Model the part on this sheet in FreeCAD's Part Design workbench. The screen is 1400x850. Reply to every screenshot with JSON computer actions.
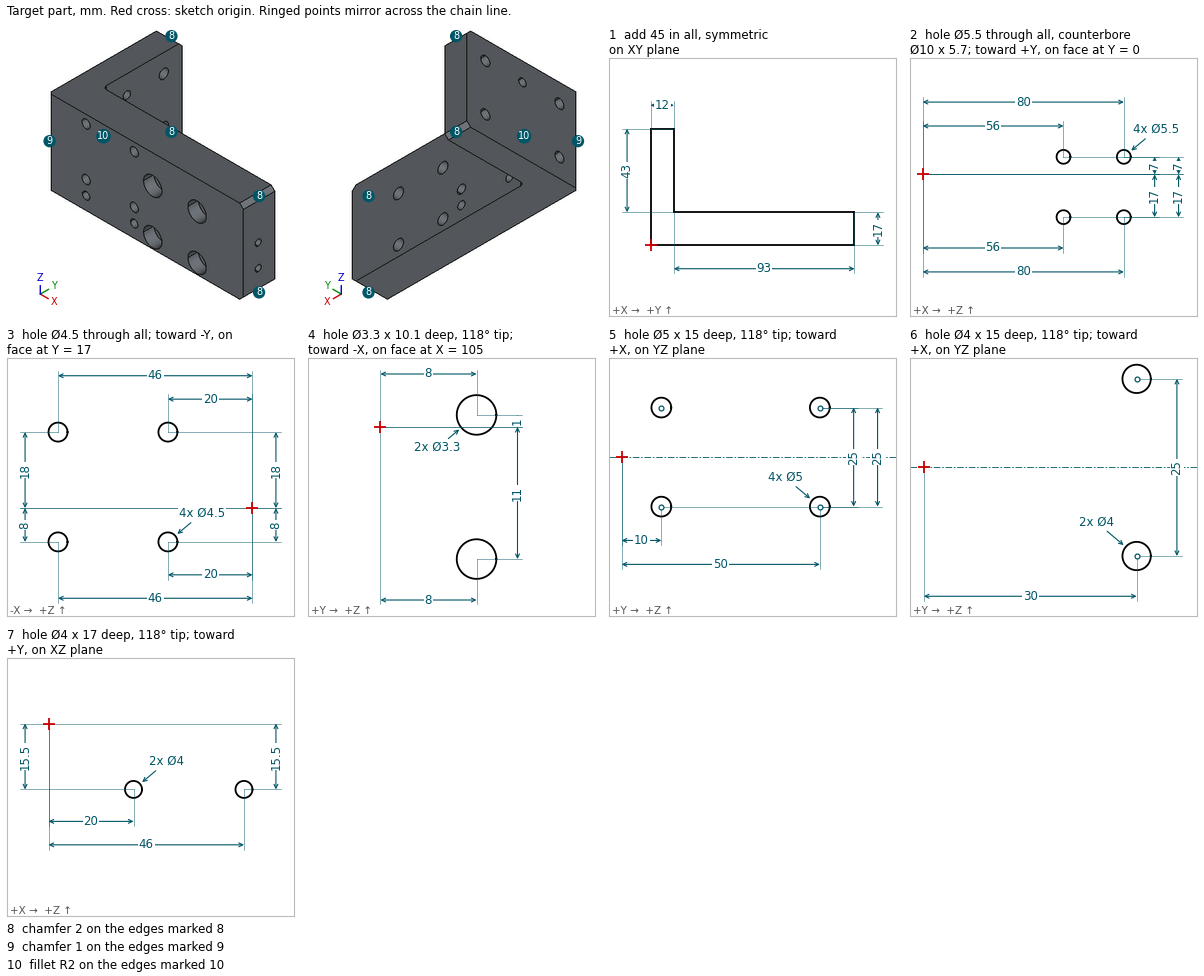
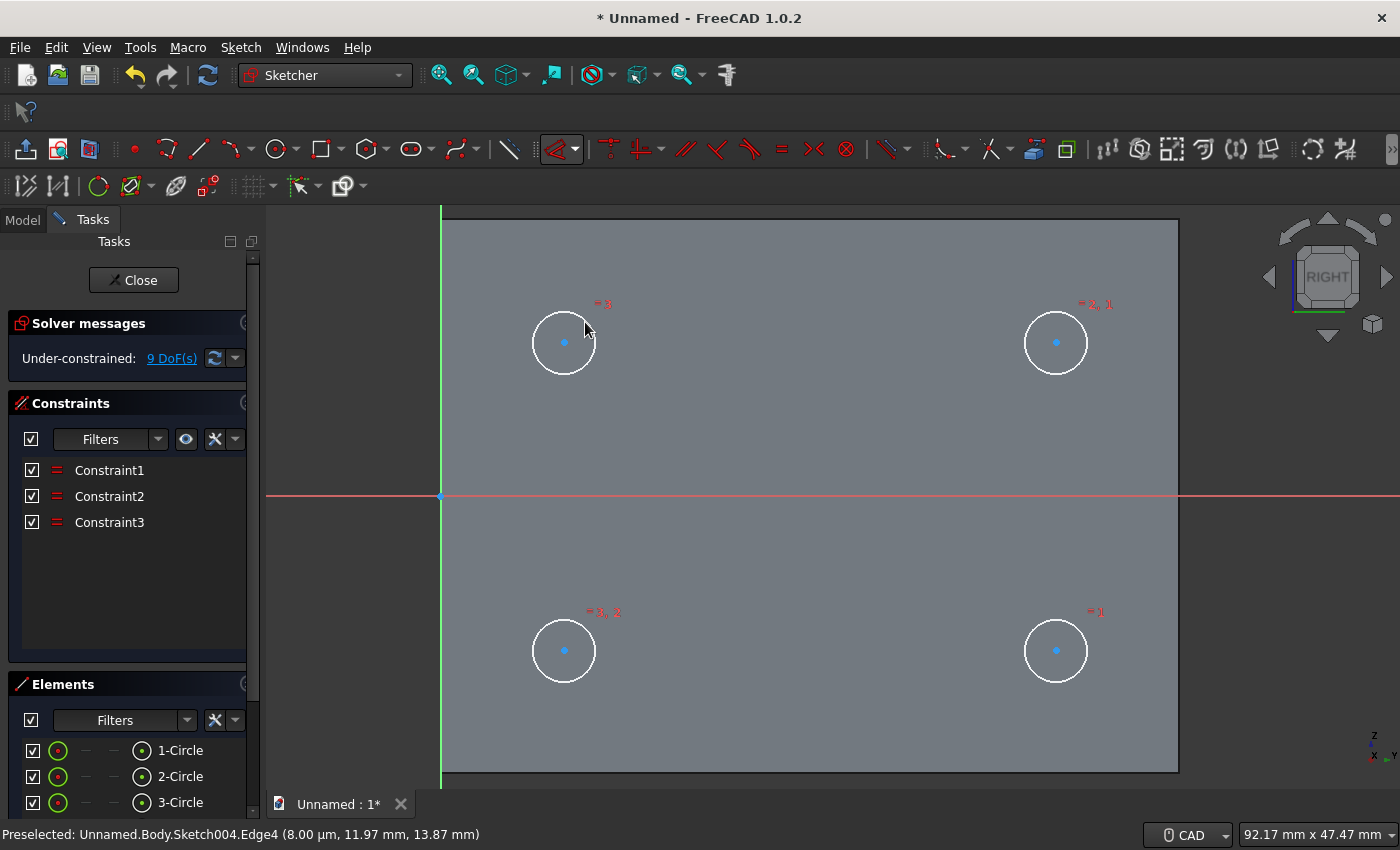
{"action": "left_click", "coordinate": [1056, 651]}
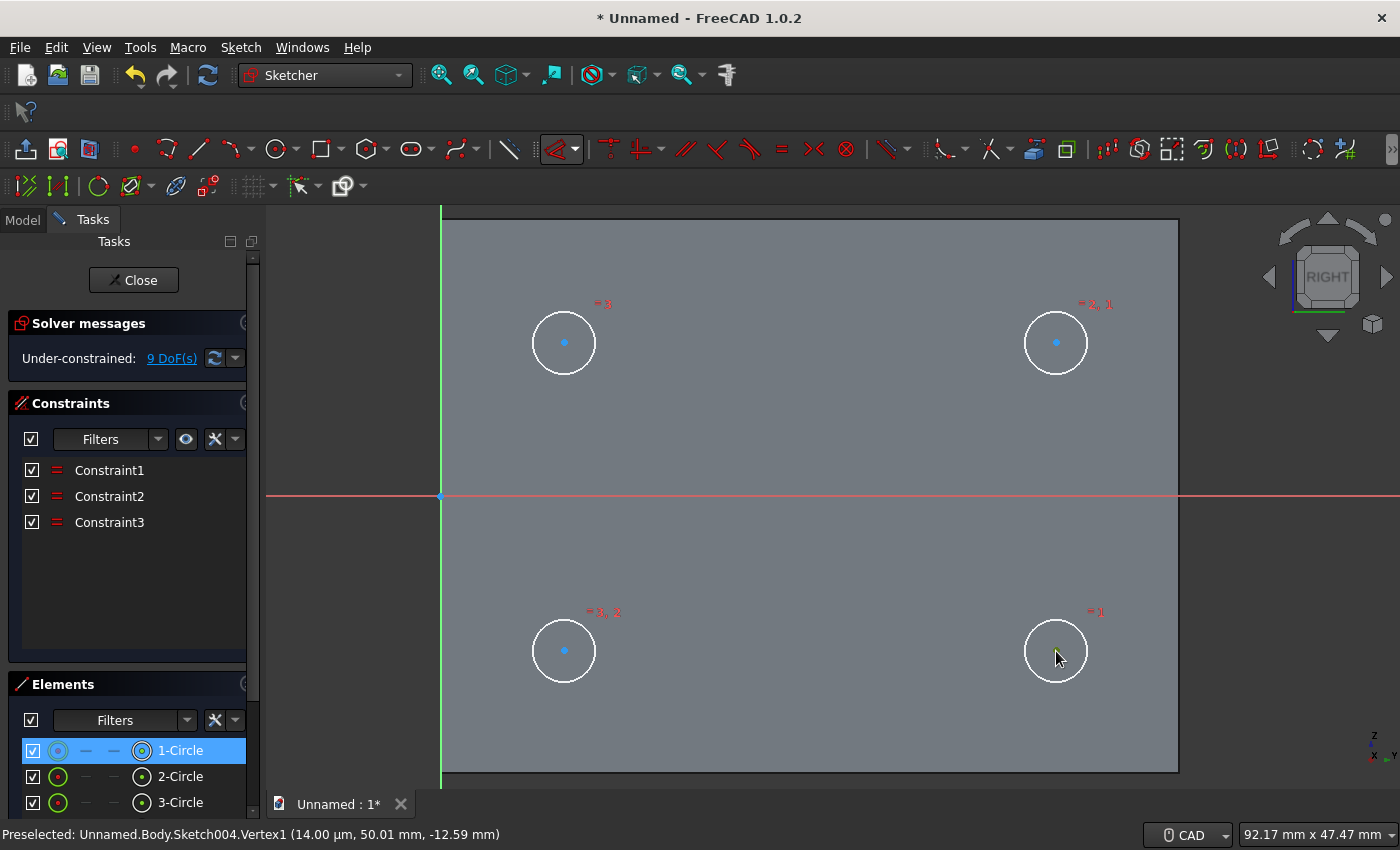
{"action": "left_click", "coordinate": [1056, 343]}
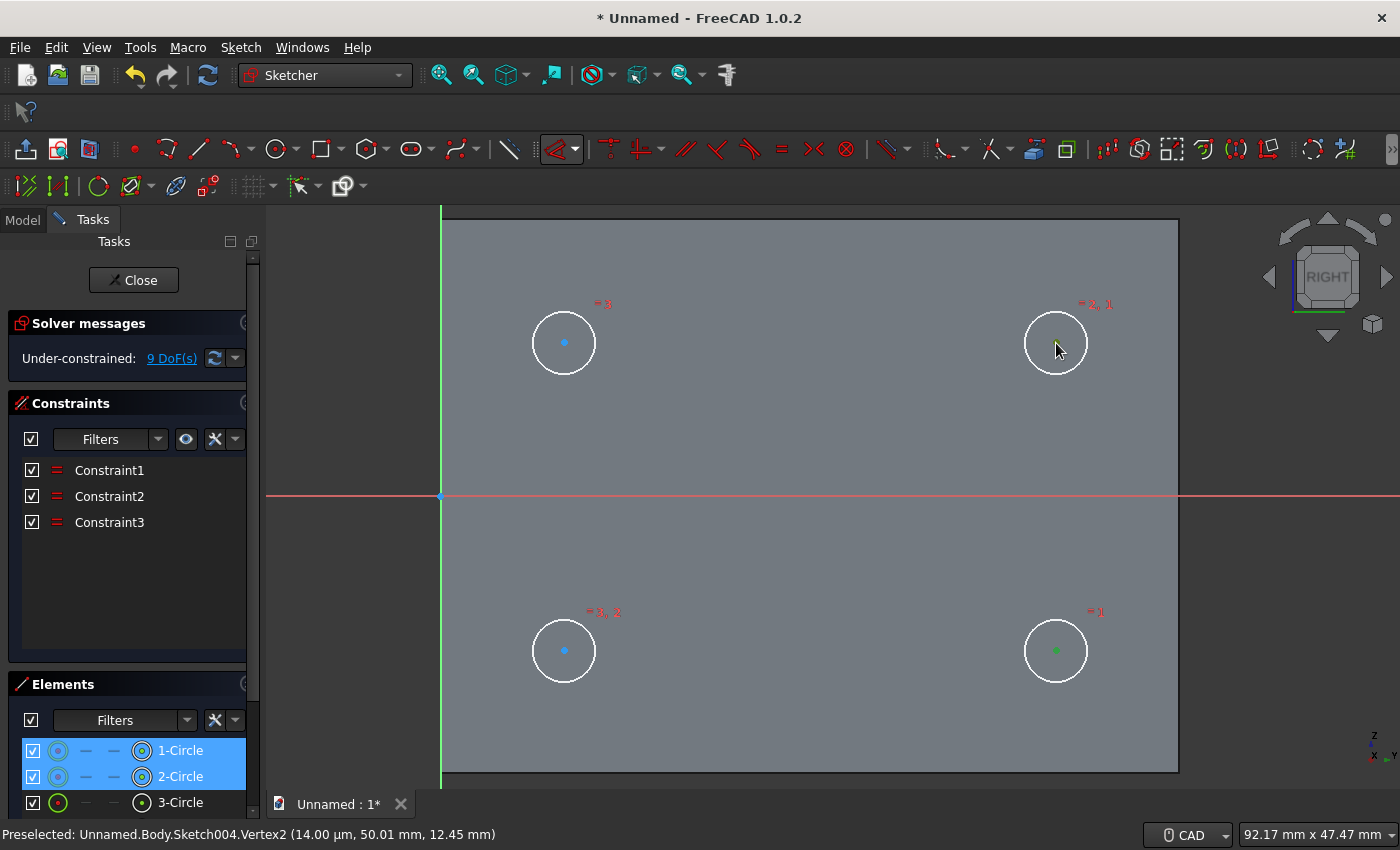
{"action": "left_click", "coordinate": [361, 496]}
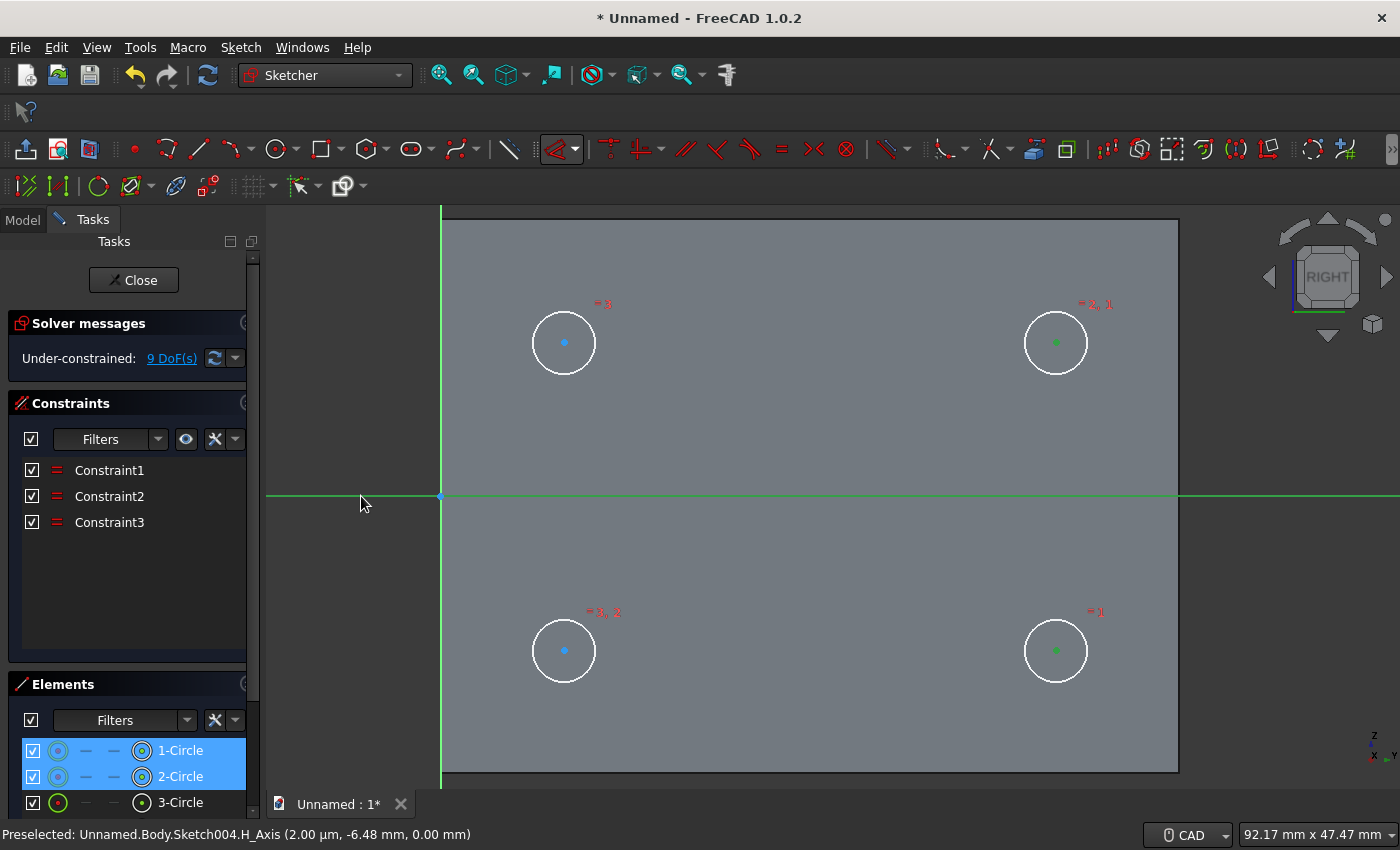
{"action": "key", "text": "s"}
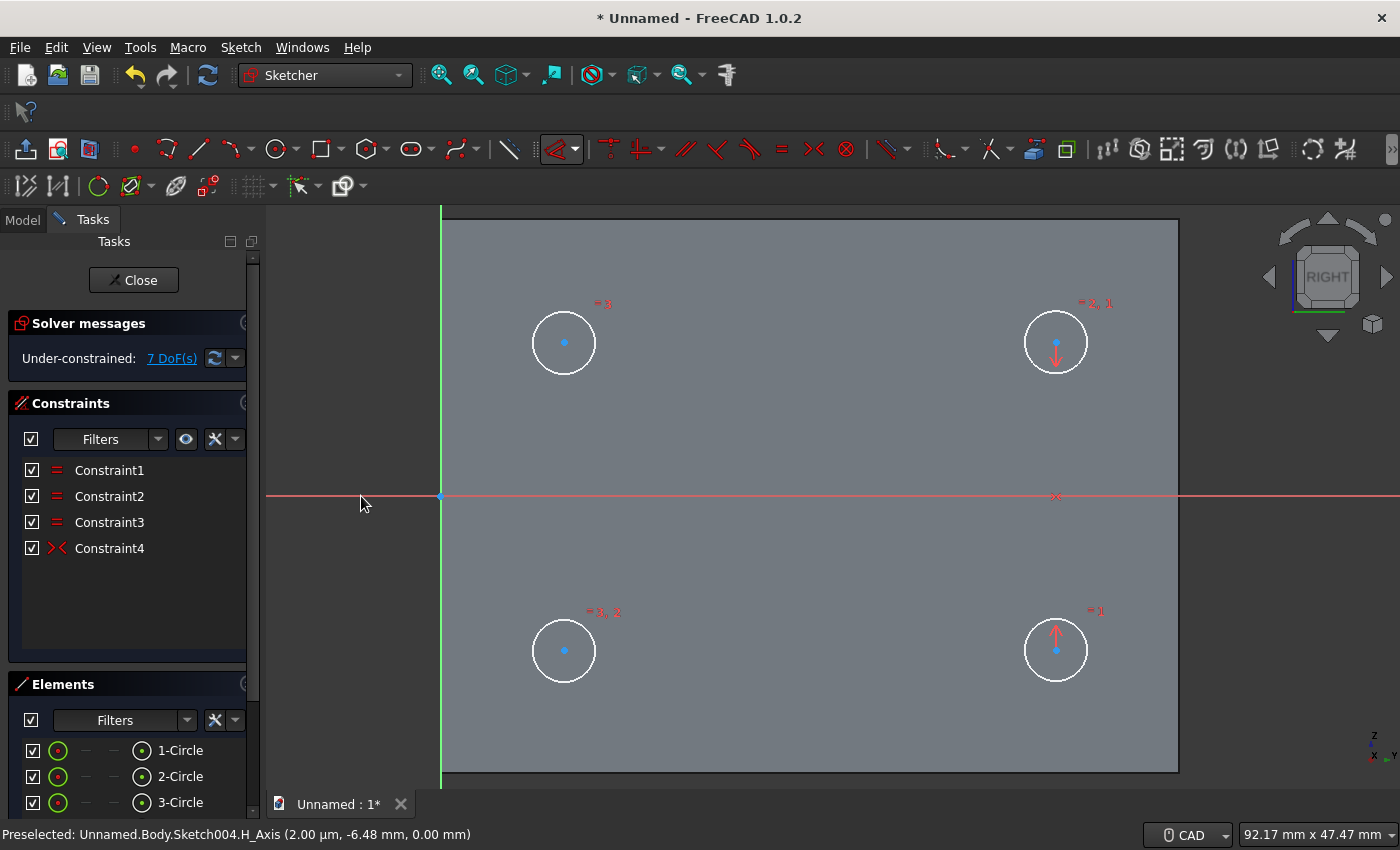
{"action": "left_click", "coordinate": [564, 651]}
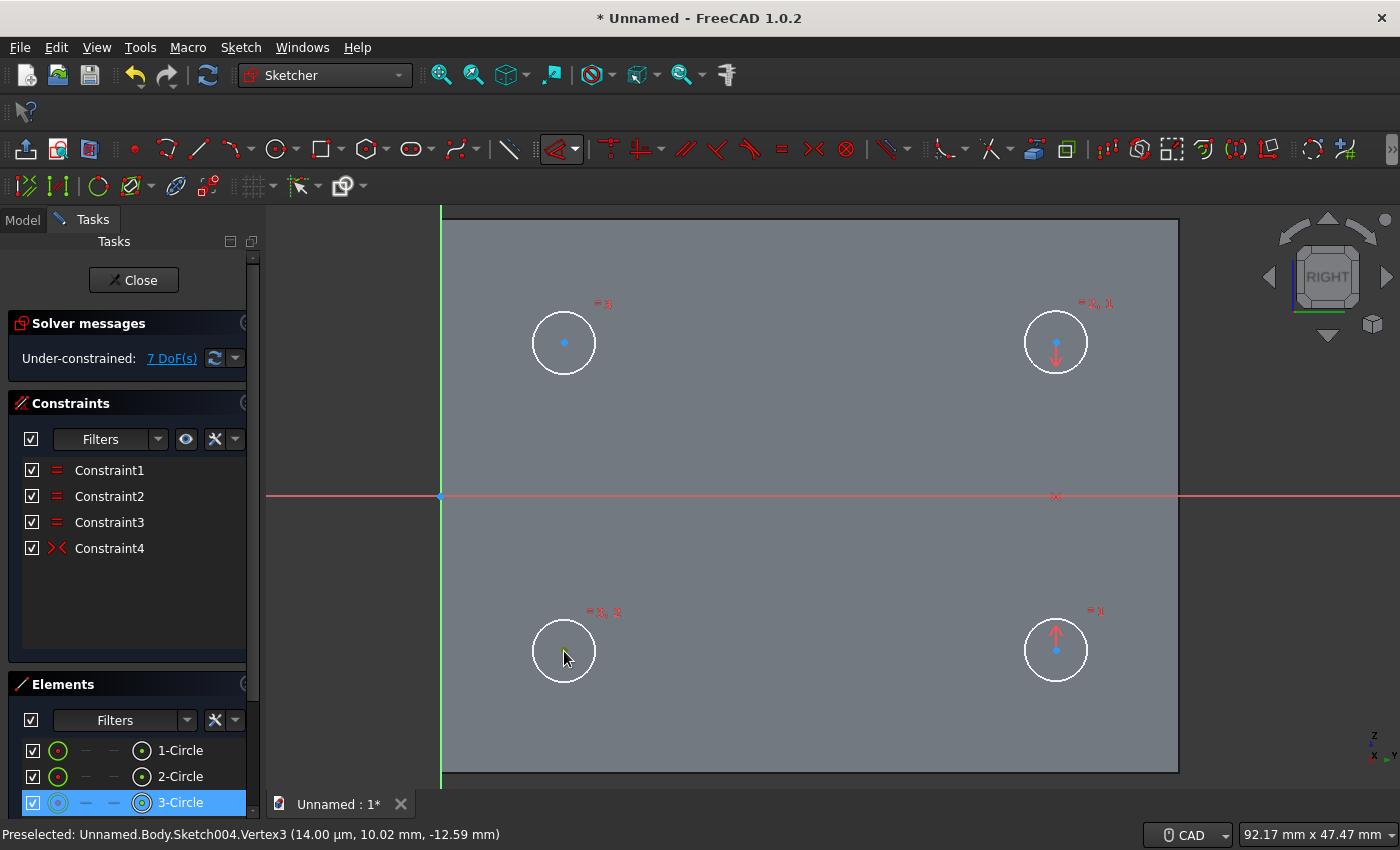
{"action": "left_click", "coordinate": [564, 343]}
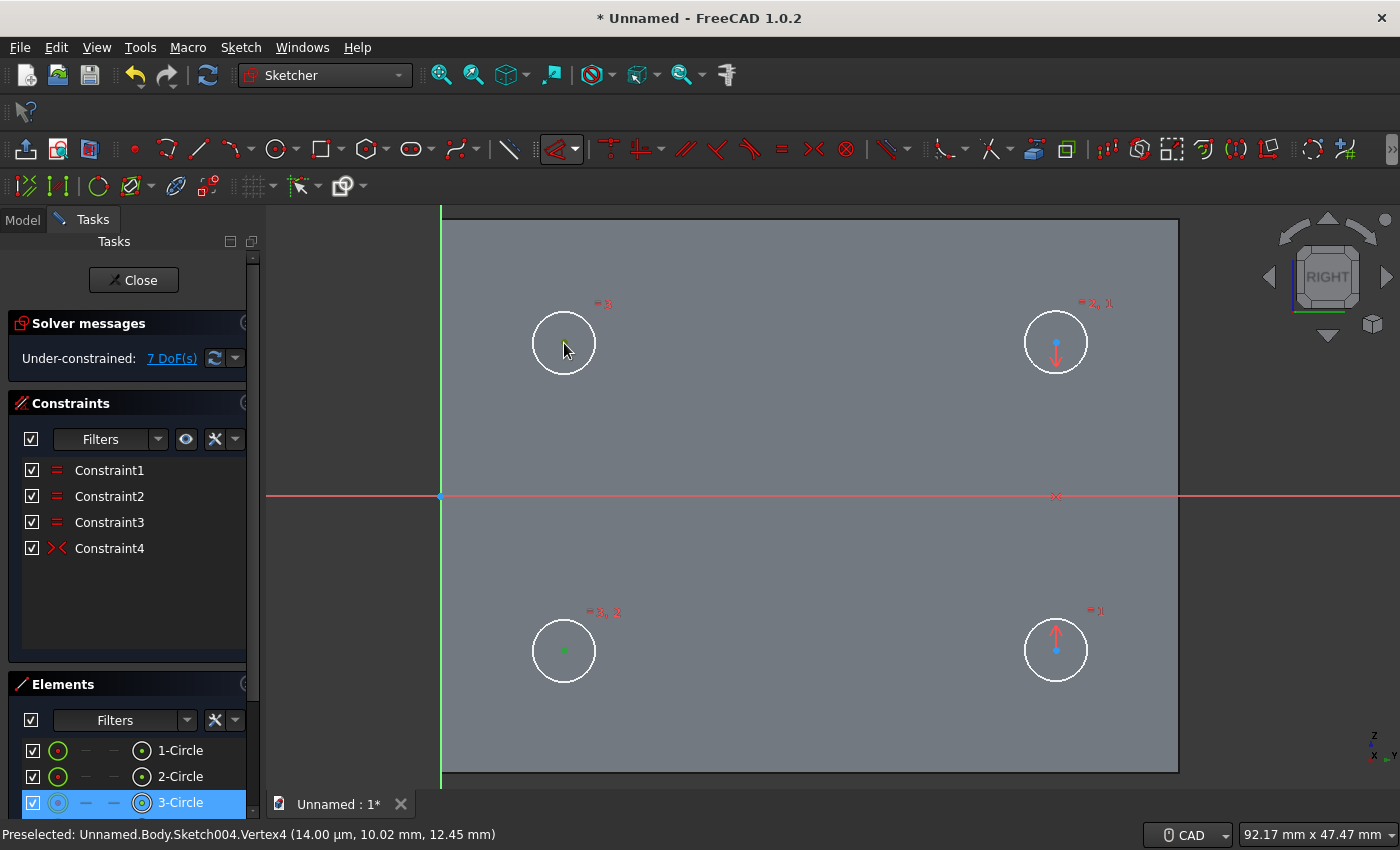
{"action": "left_click", "coordinate": [361, 496]}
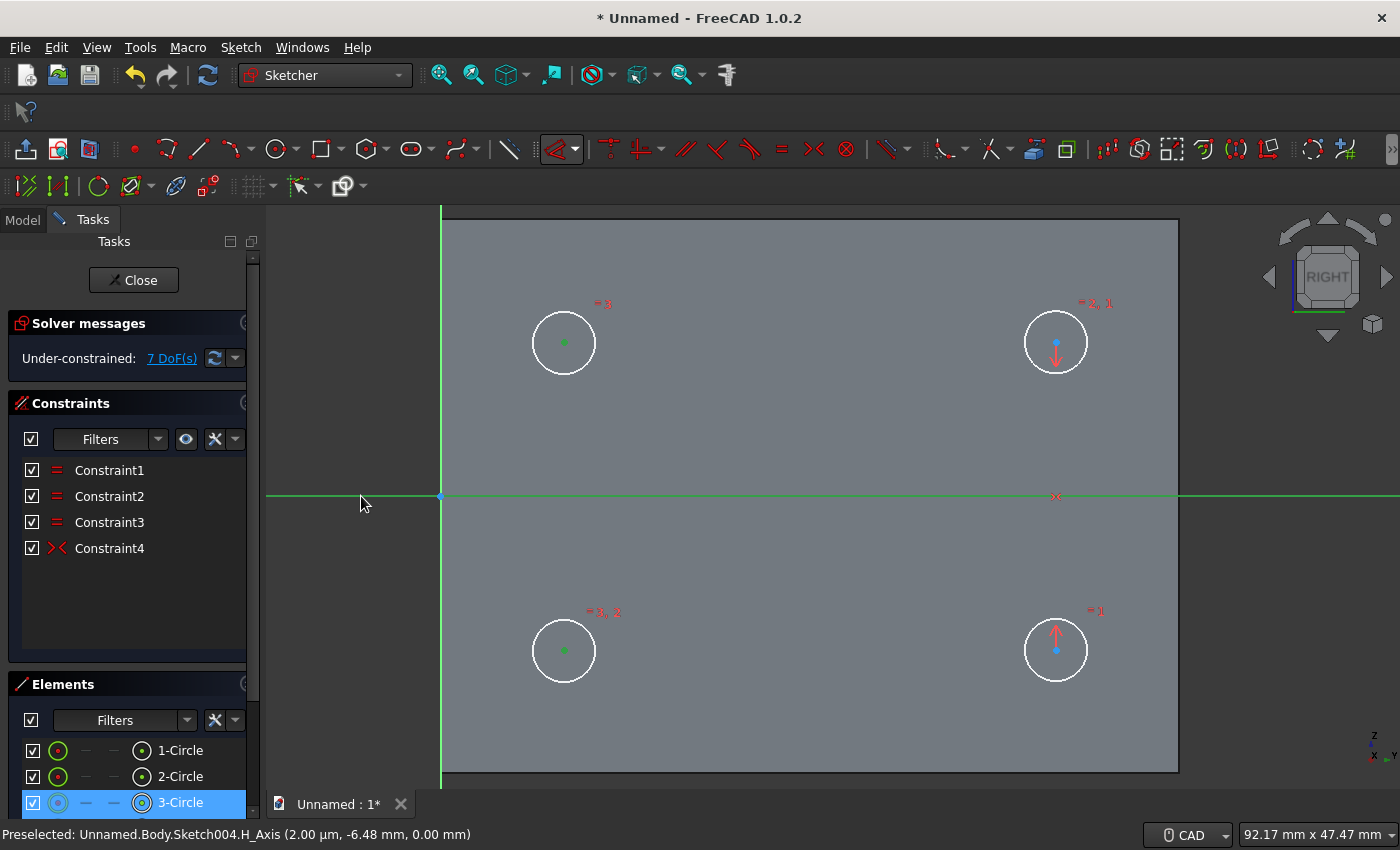
{"action": "left_click", "coordinate": [814, 150]}